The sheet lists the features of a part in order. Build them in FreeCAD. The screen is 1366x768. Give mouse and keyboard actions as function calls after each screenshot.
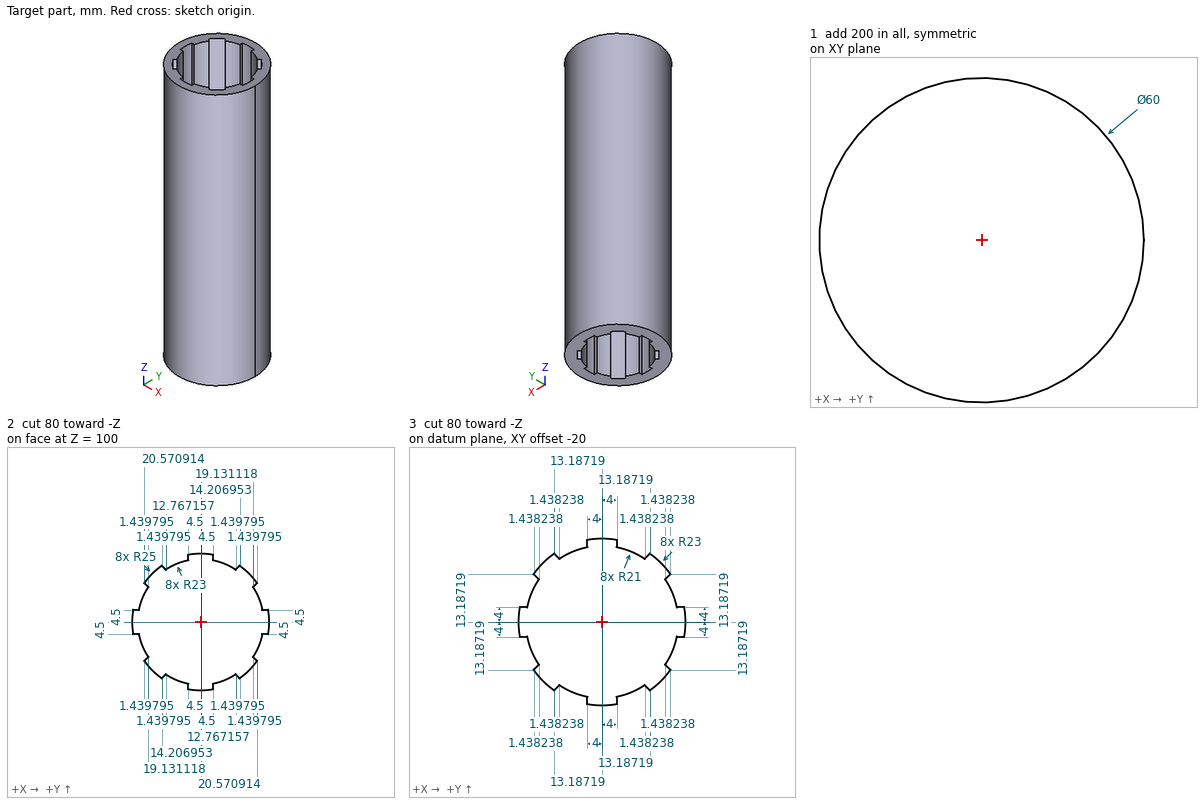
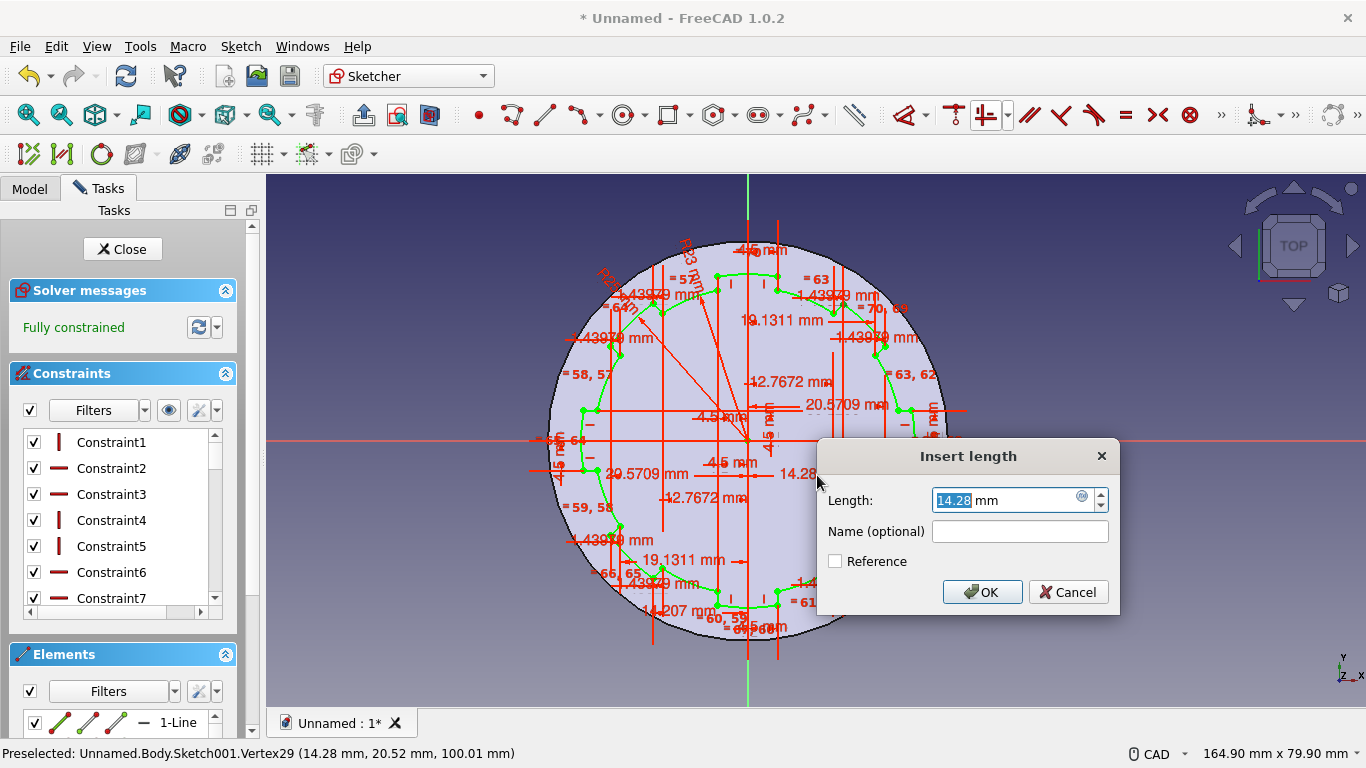
text(14.206953)
key(Return)
key(Escape)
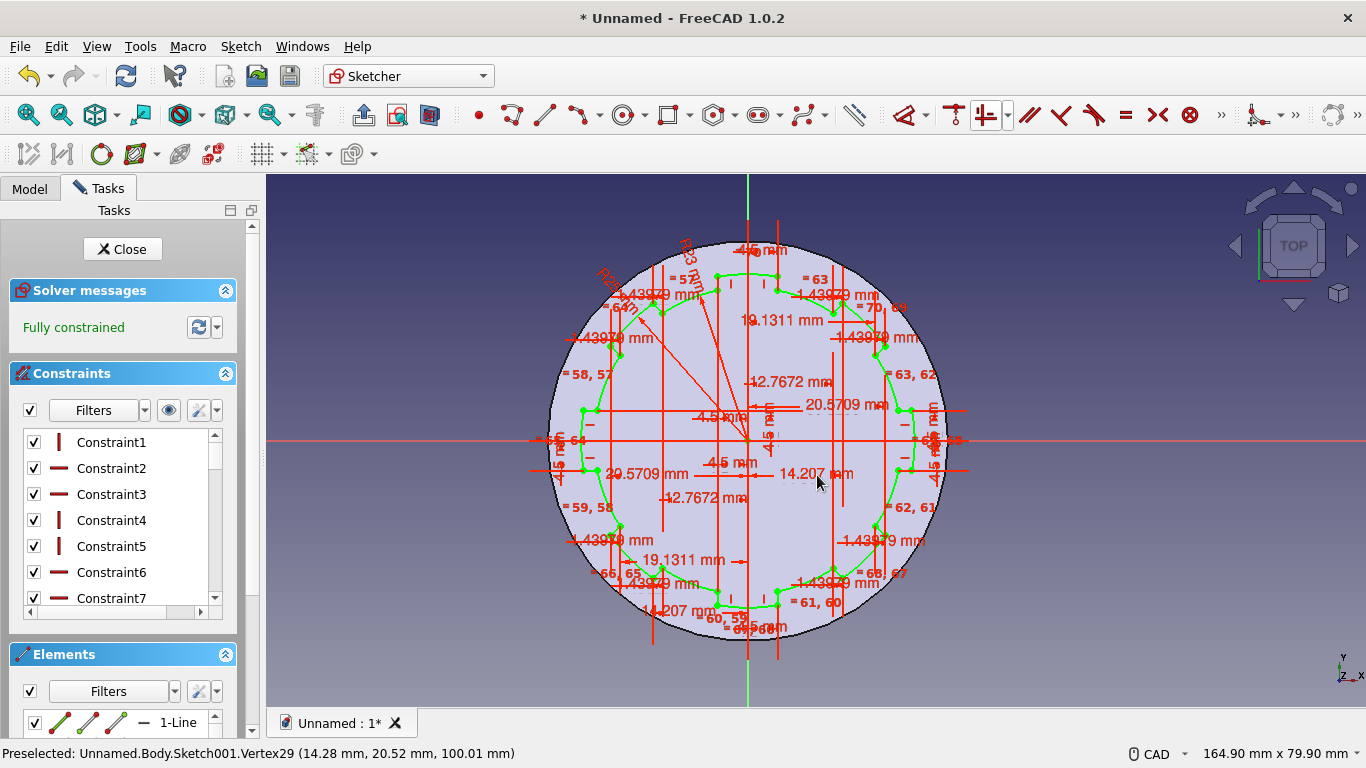
click(123, 249)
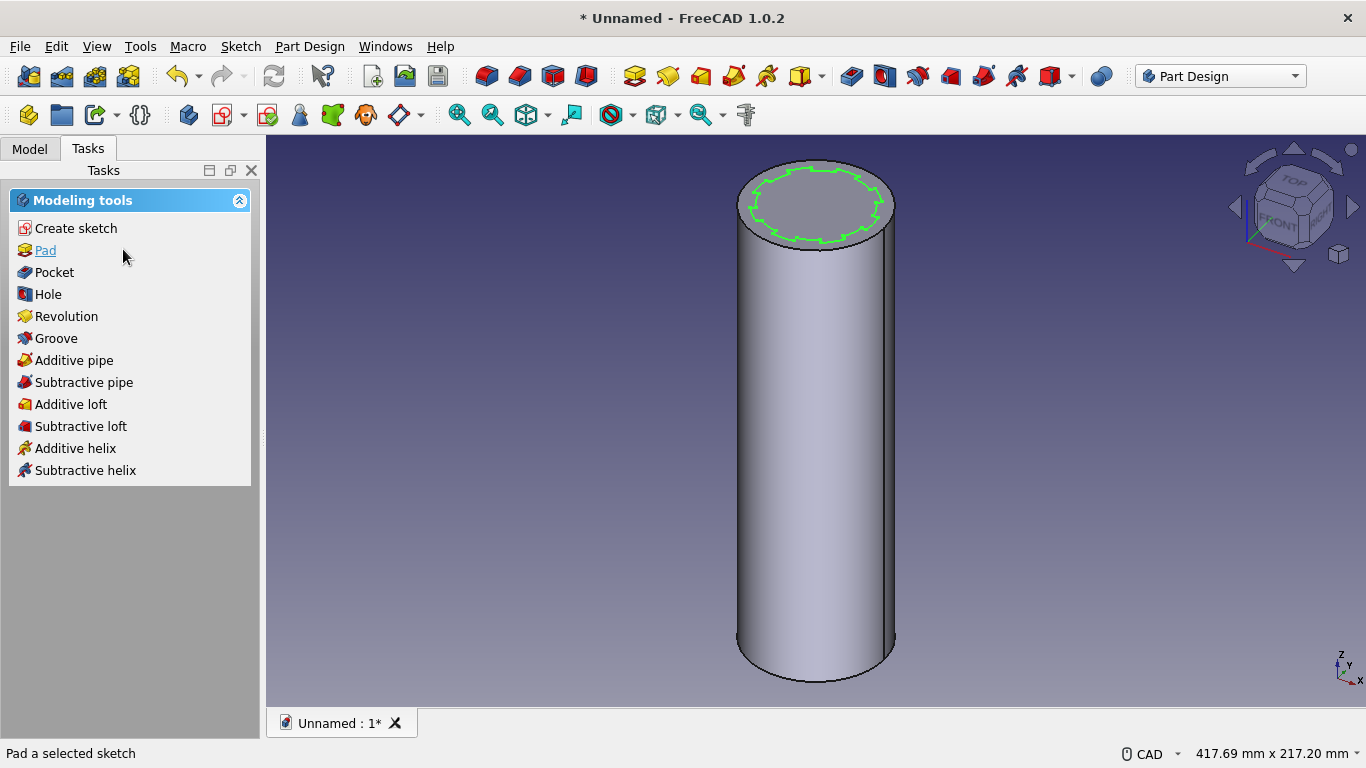
click(852, 76)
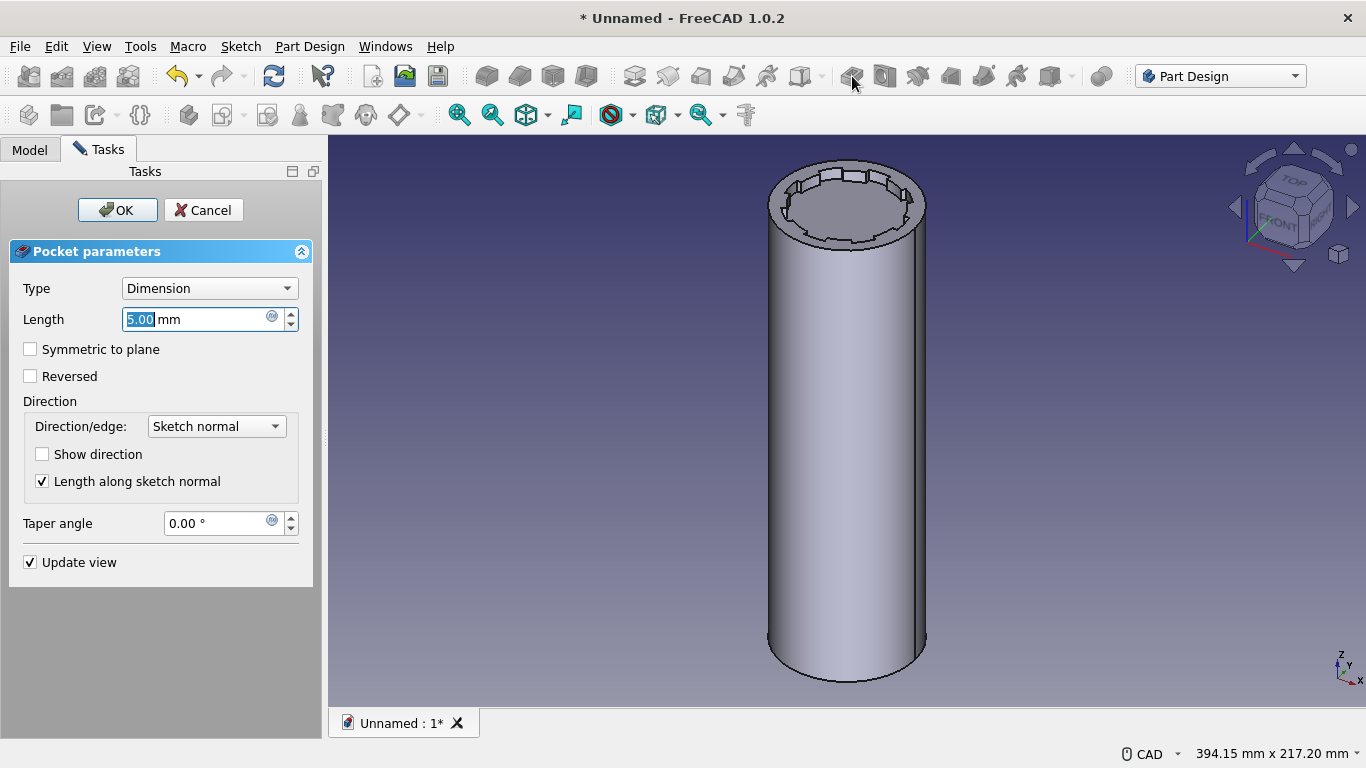
text(80)
key(Tab)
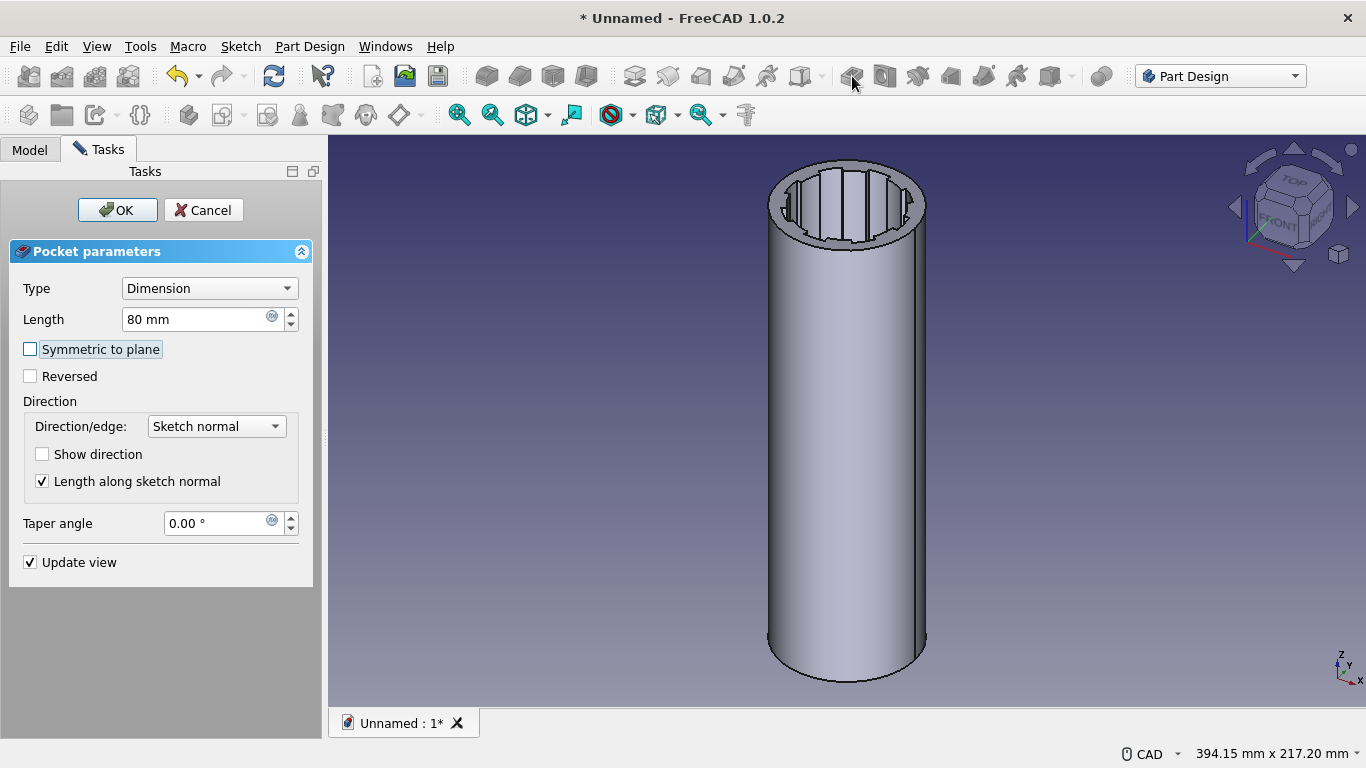
click(118, 210)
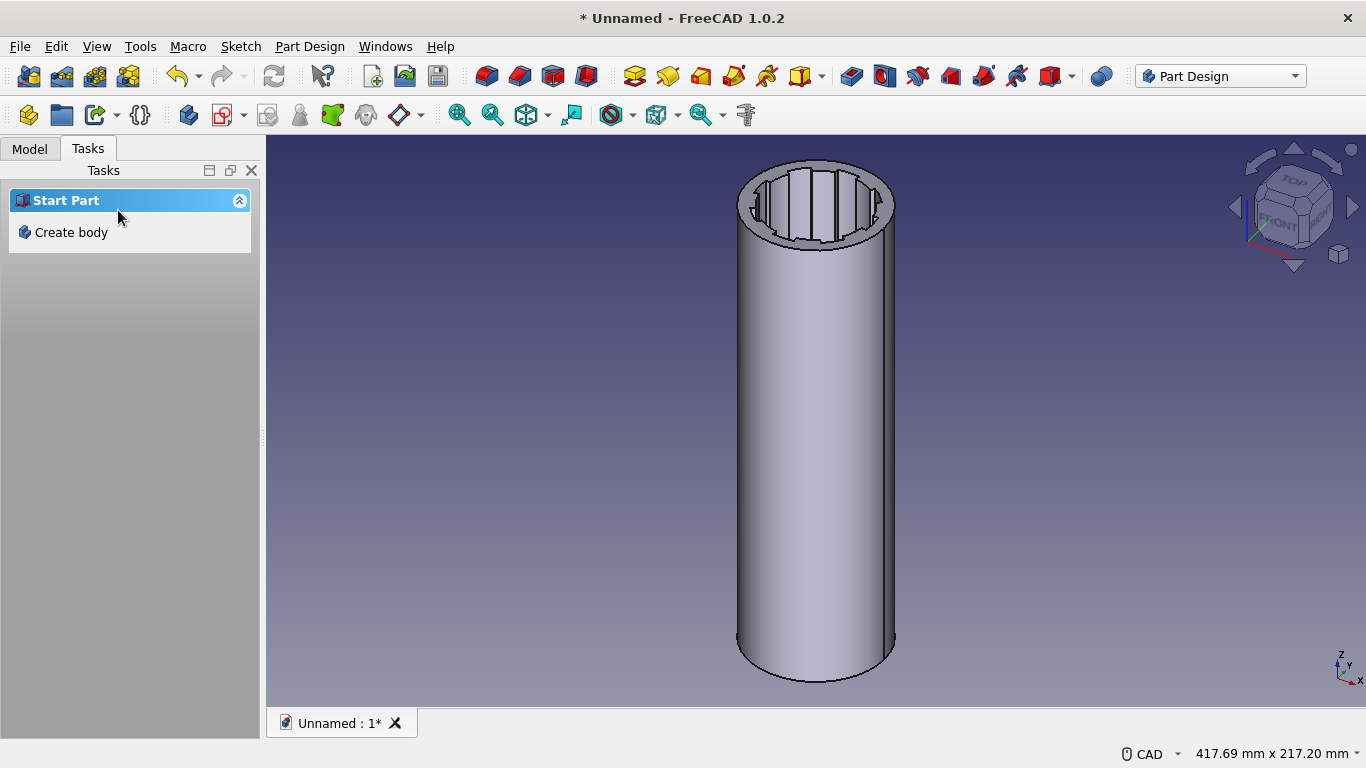
click(30, 148)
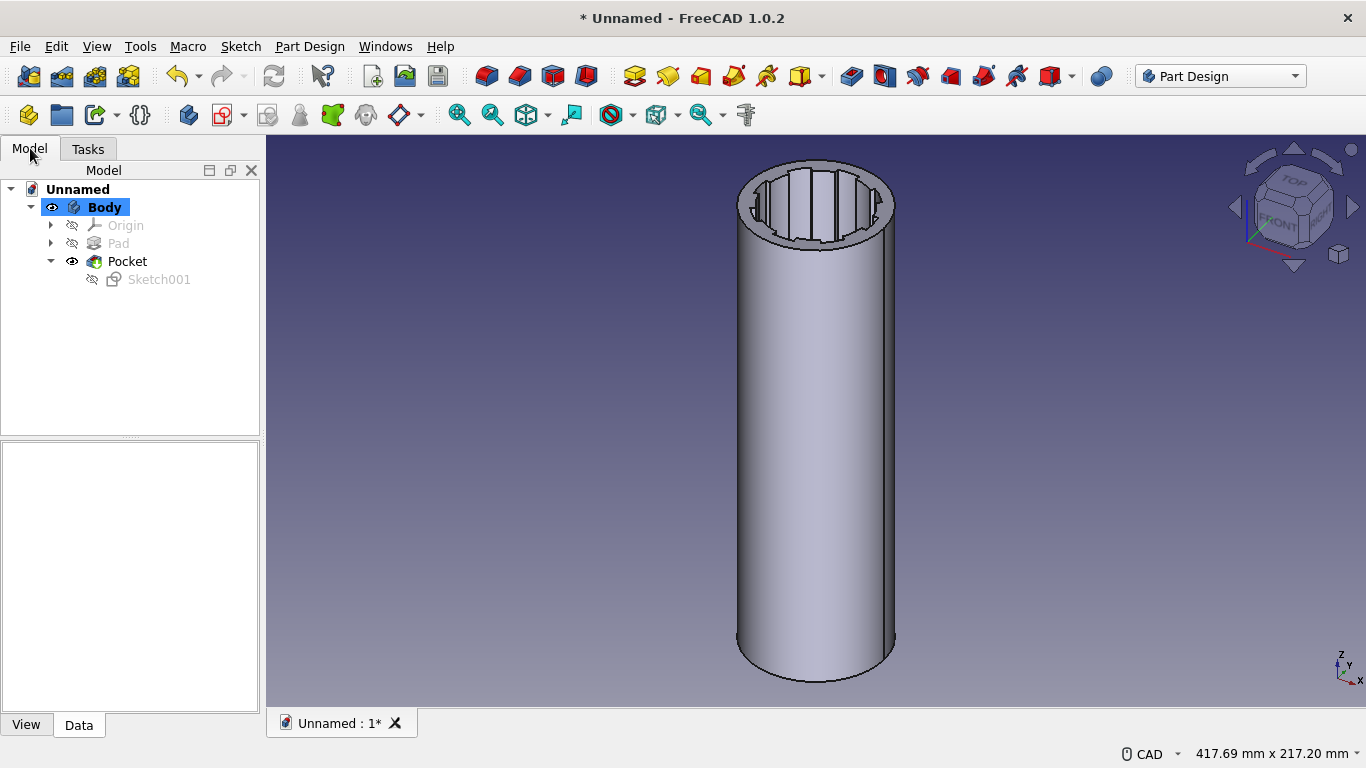
click(51, 225)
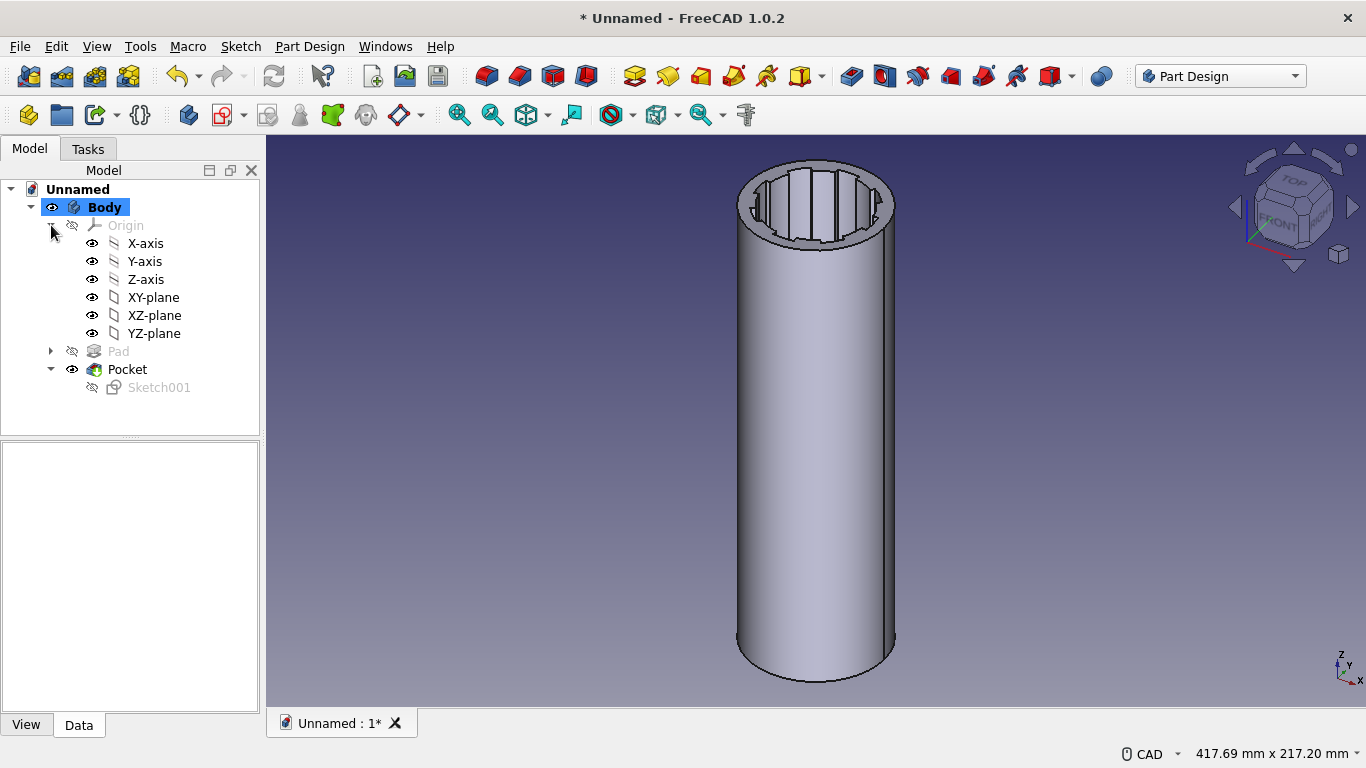
click(137, 297)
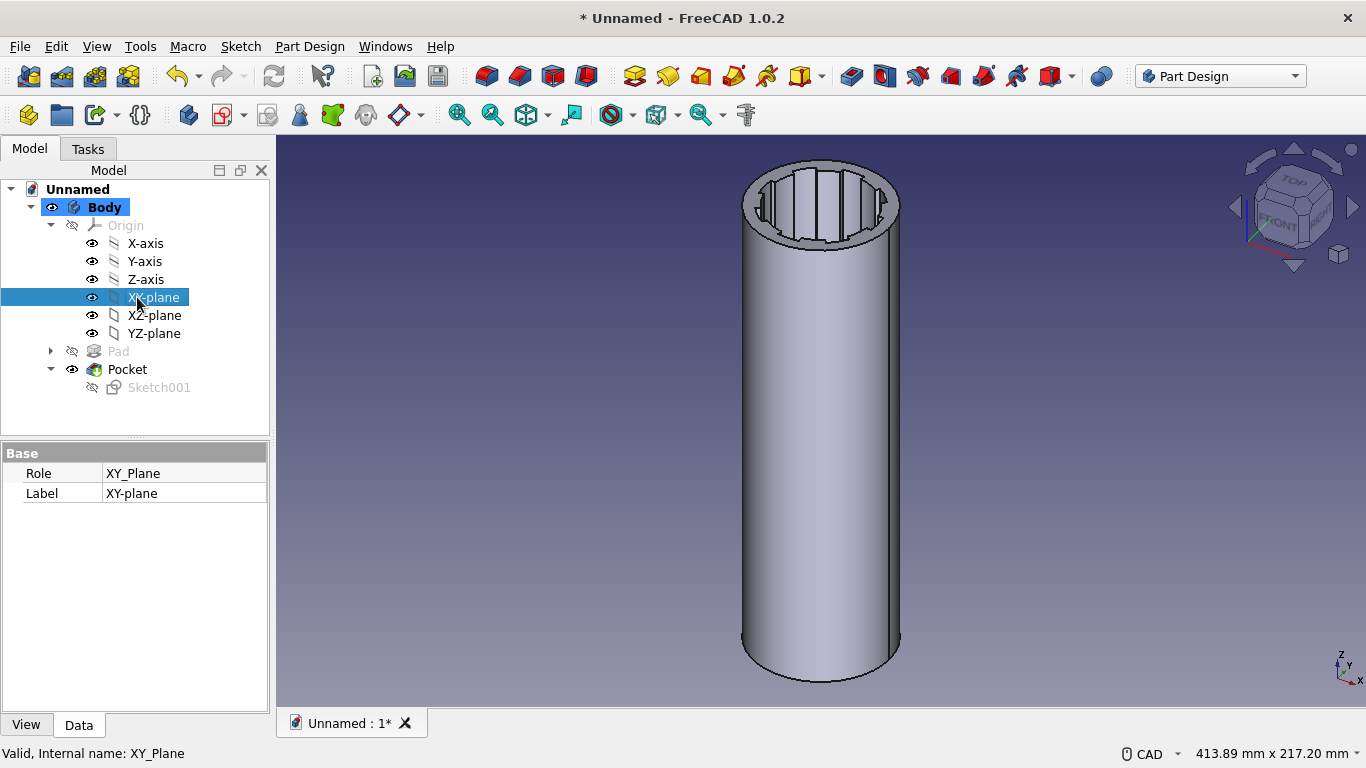
click(398, 116)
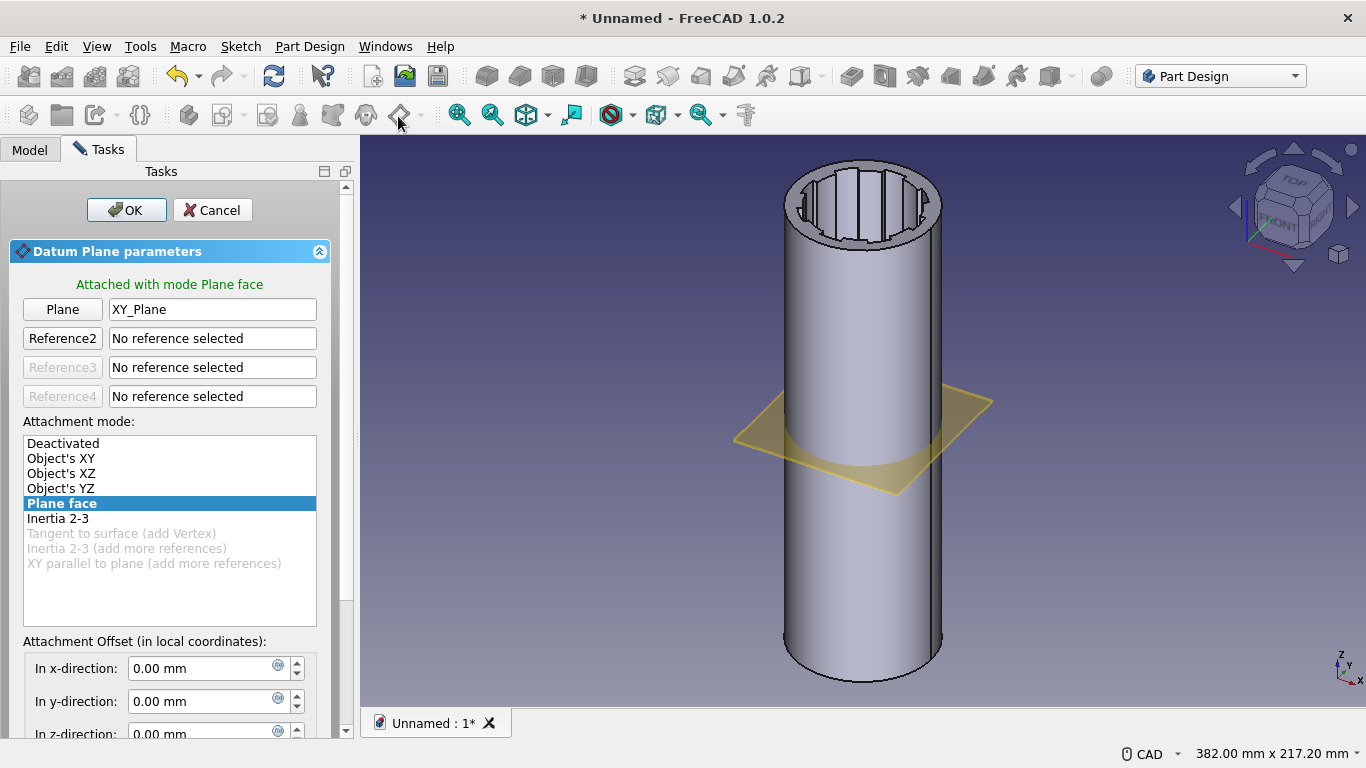
scroll(346, 460, down, 2)